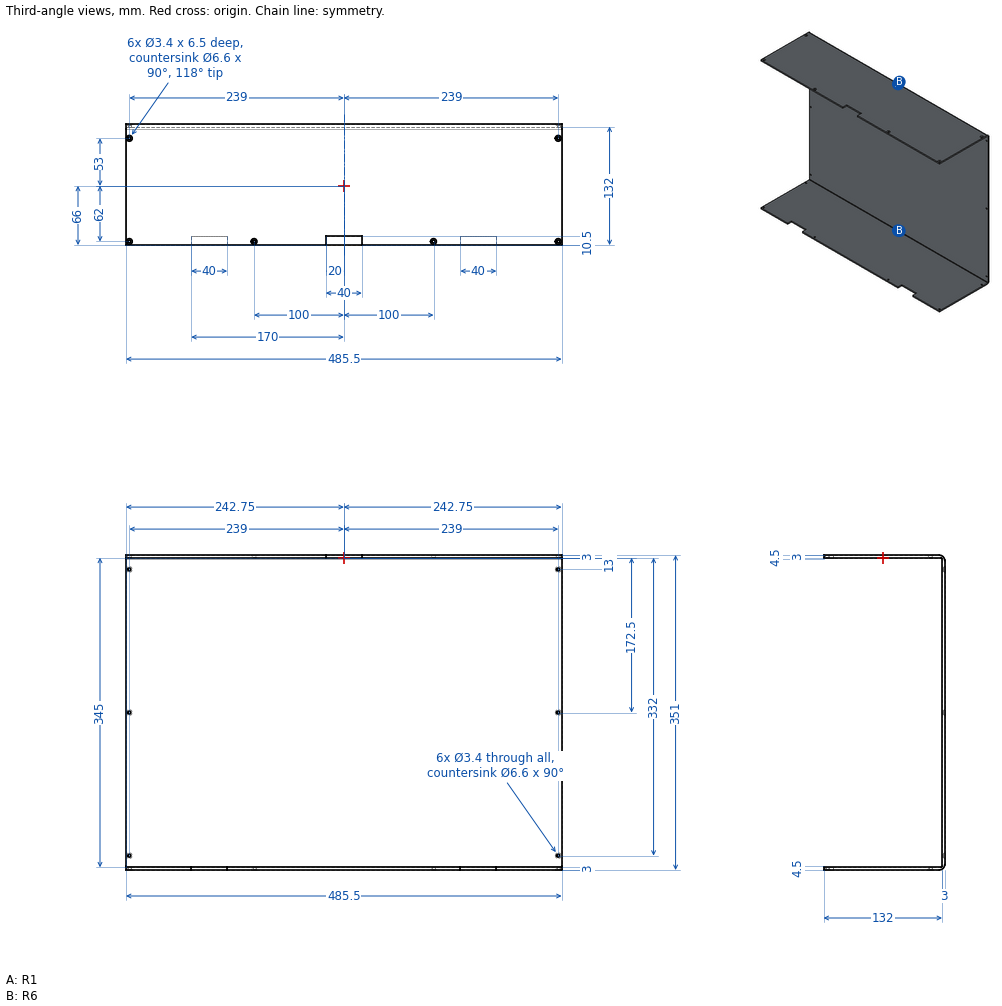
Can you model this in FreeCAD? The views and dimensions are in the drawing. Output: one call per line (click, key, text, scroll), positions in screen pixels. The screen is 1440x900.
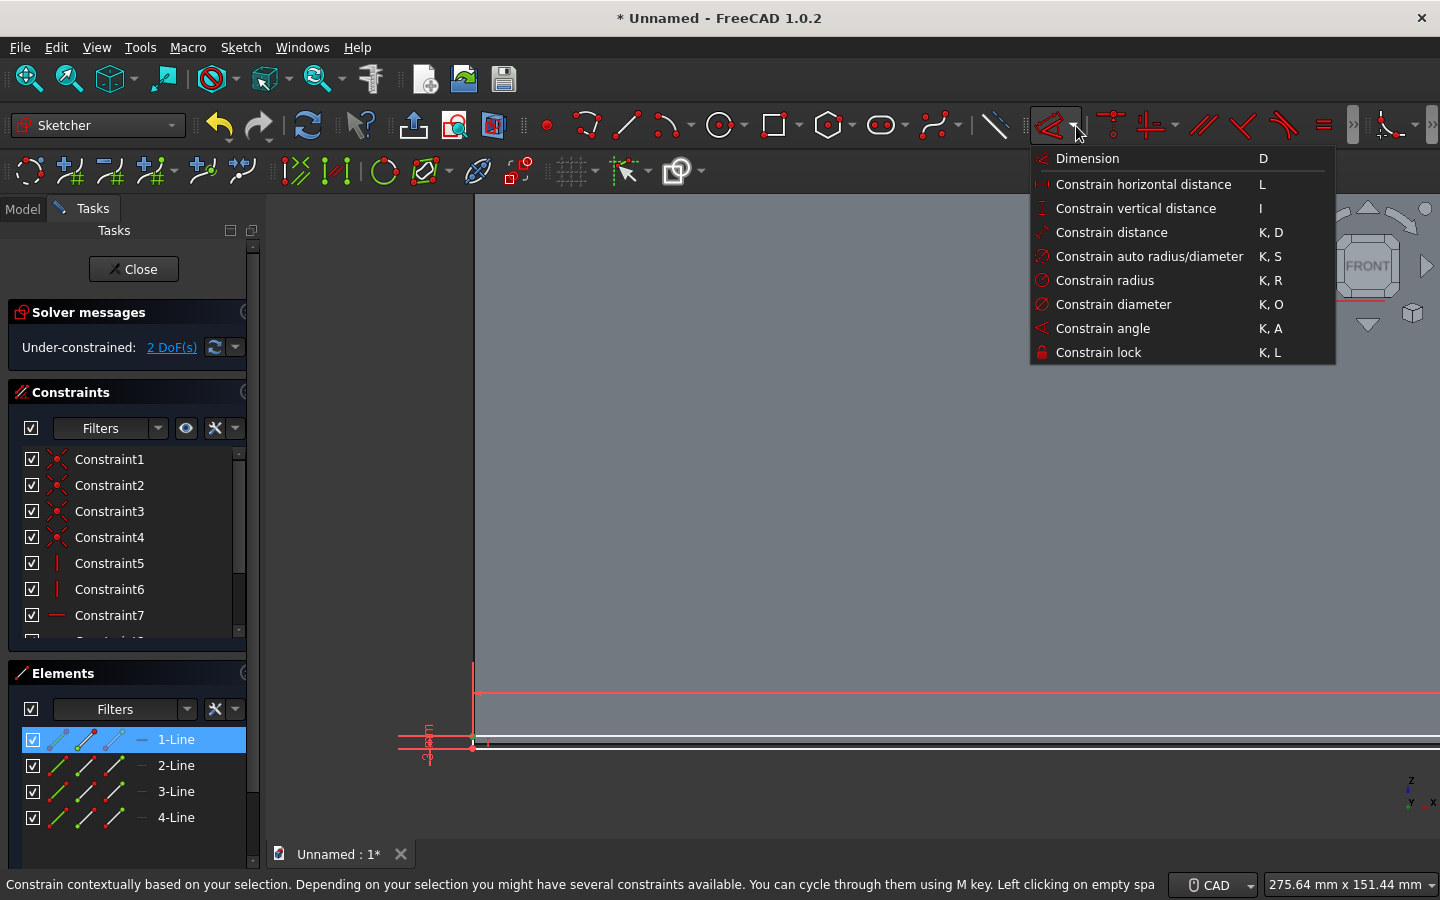
click(1183, 208)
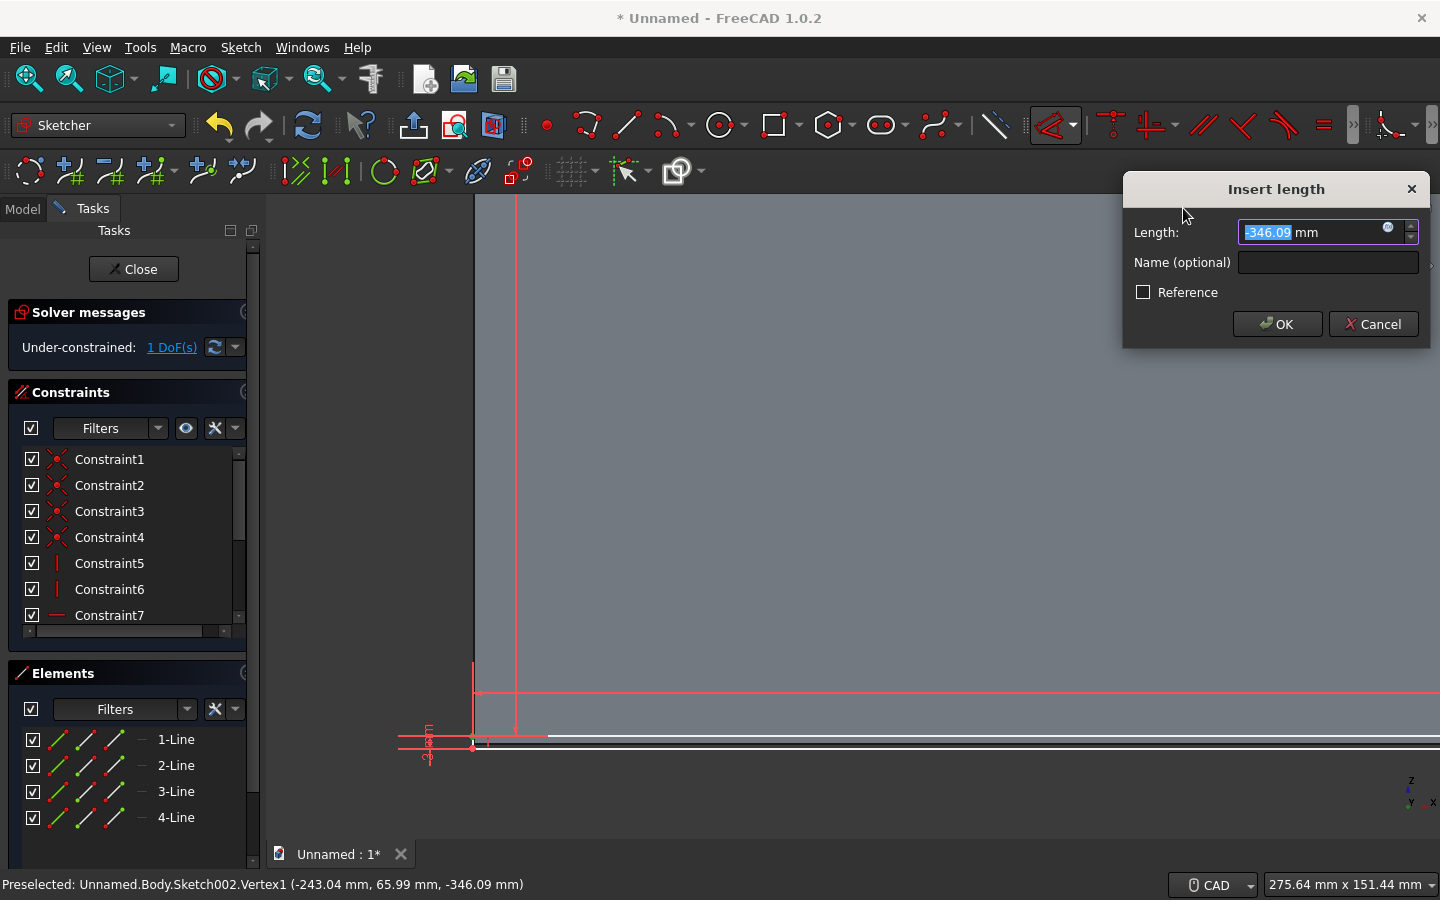
text(-345)
key(Return)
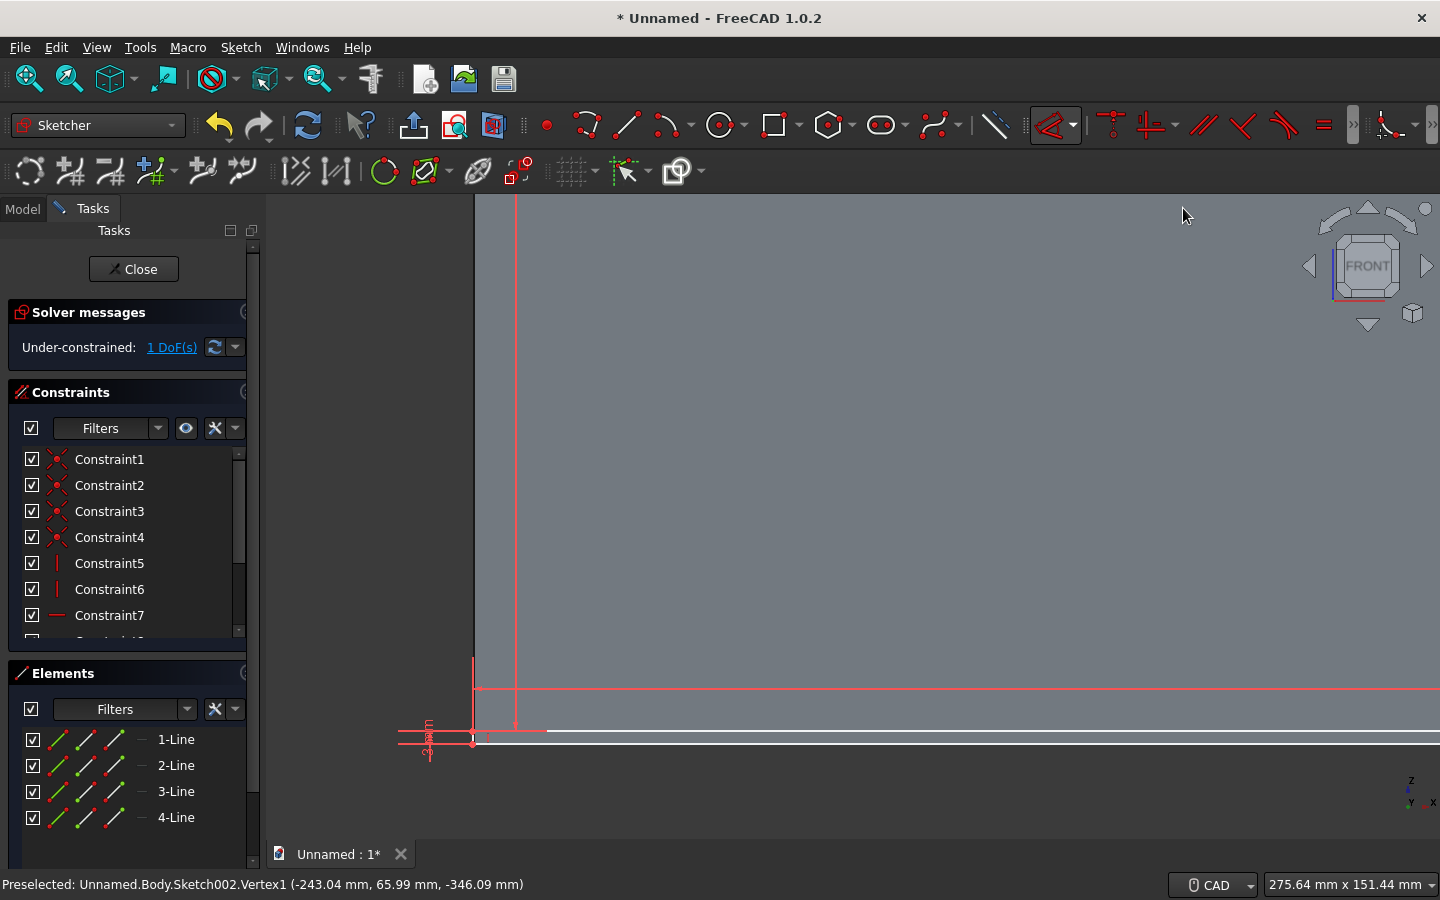
click(473, 731)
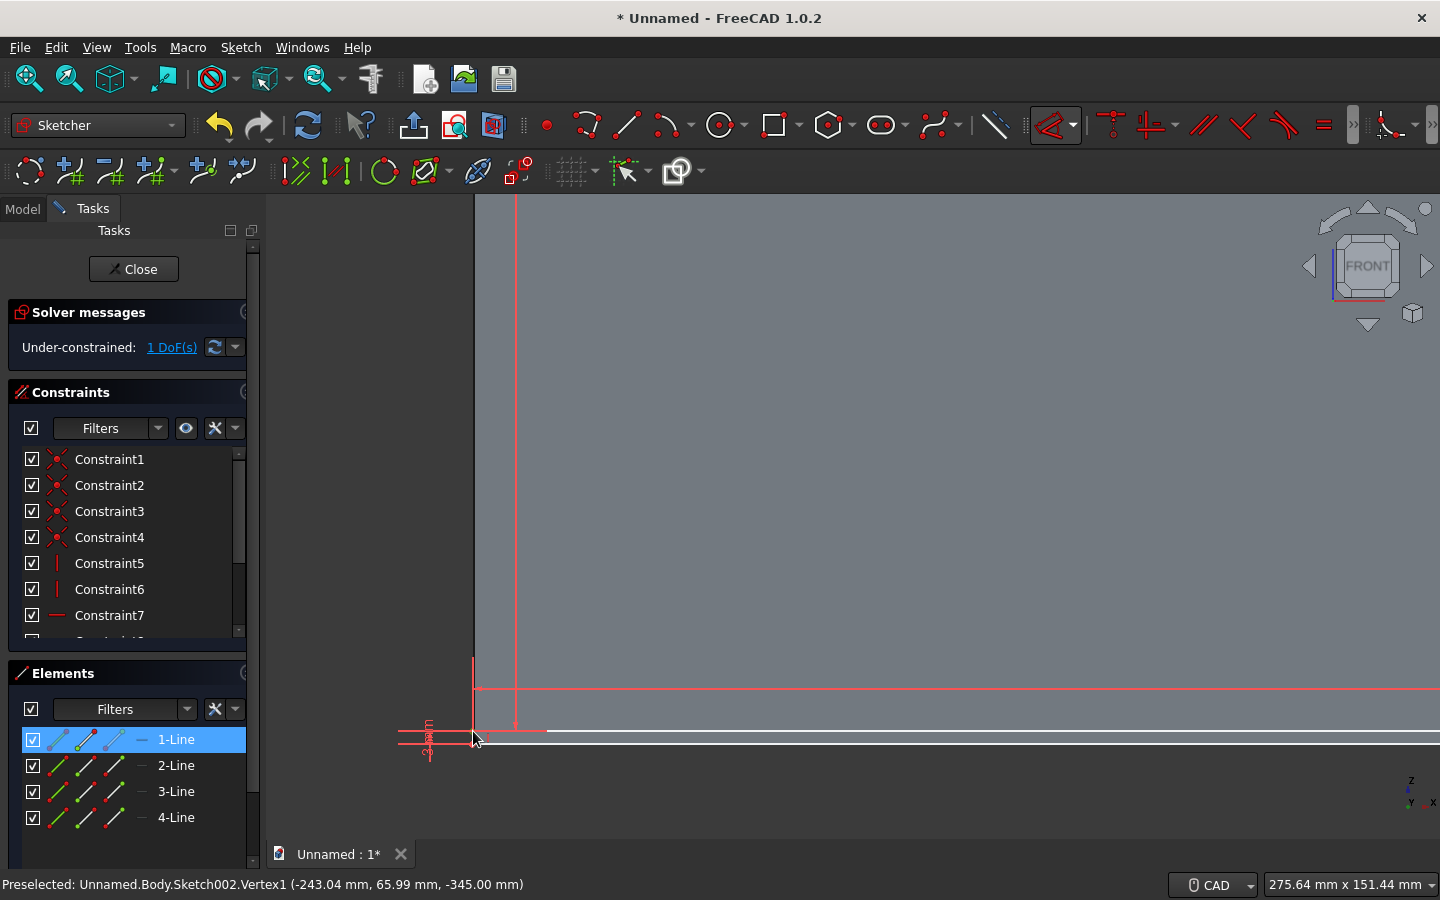
click(1076, 126)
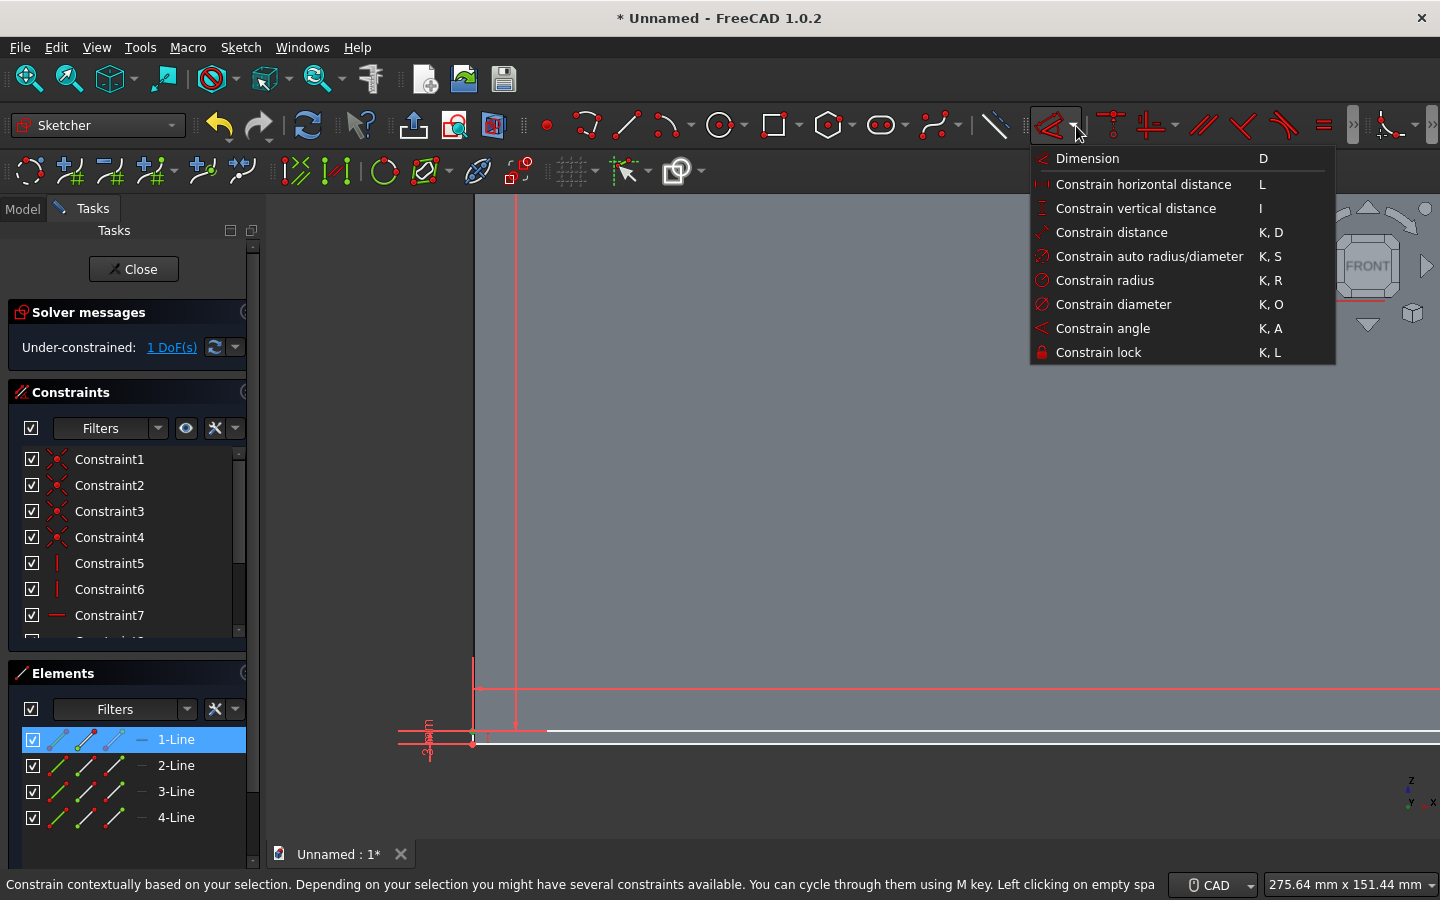
click(1183, 184)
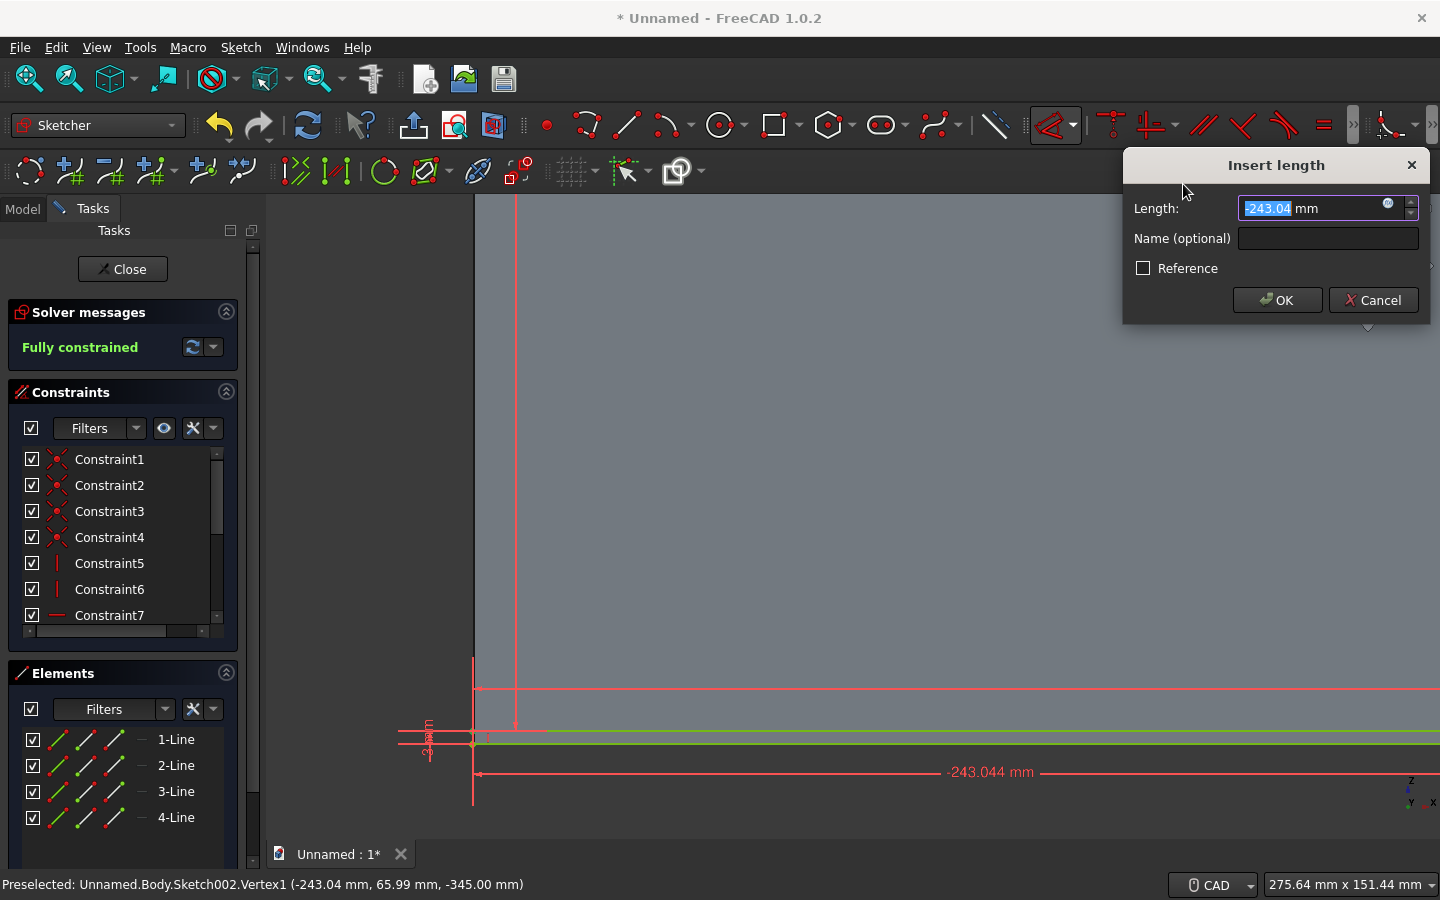
text(-242.75)
key(Return)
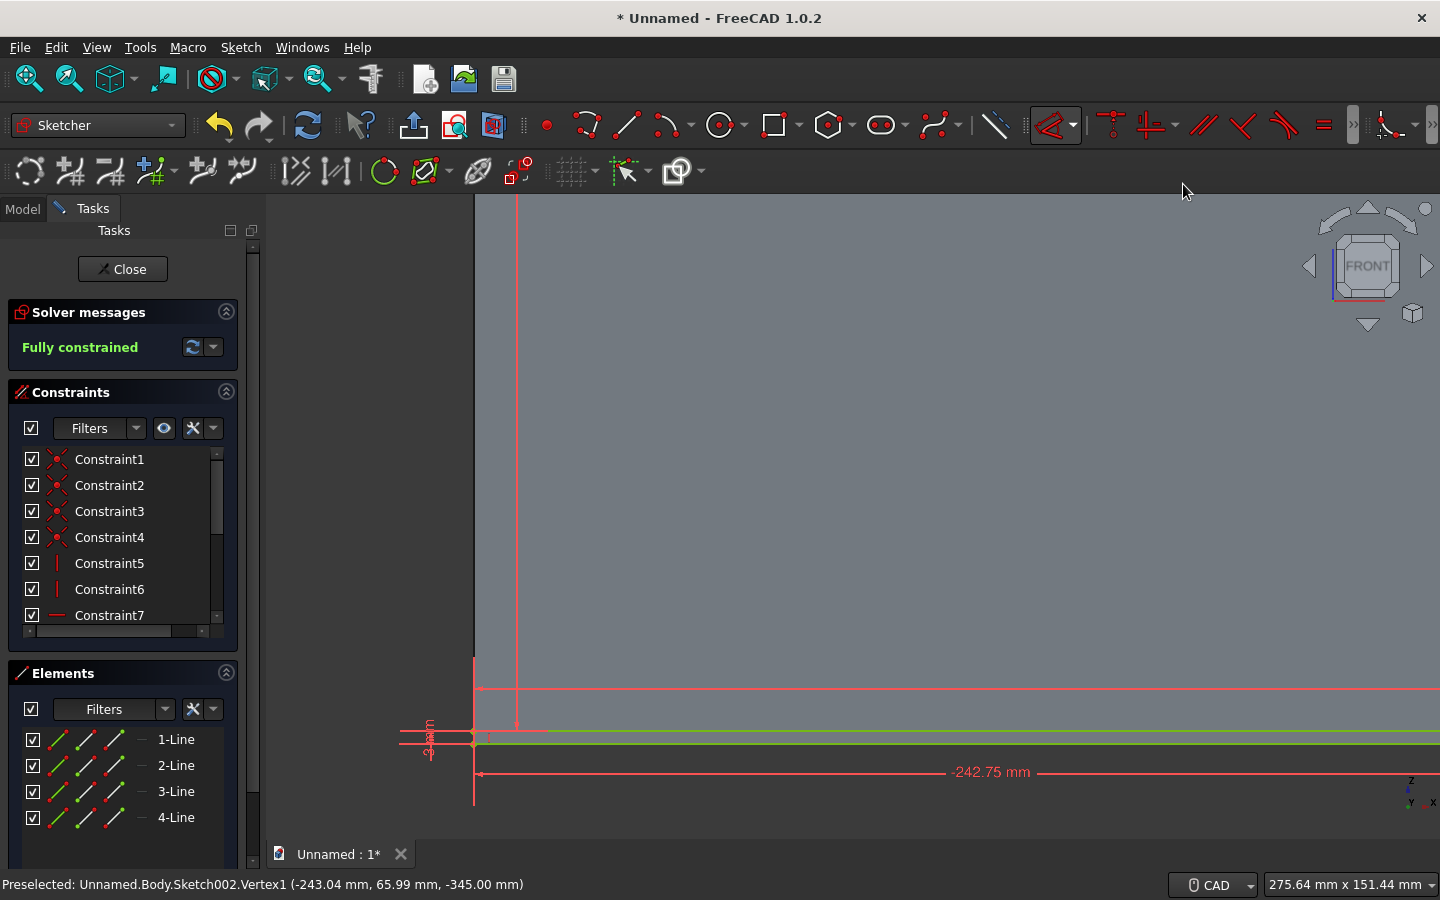
click(123, 269)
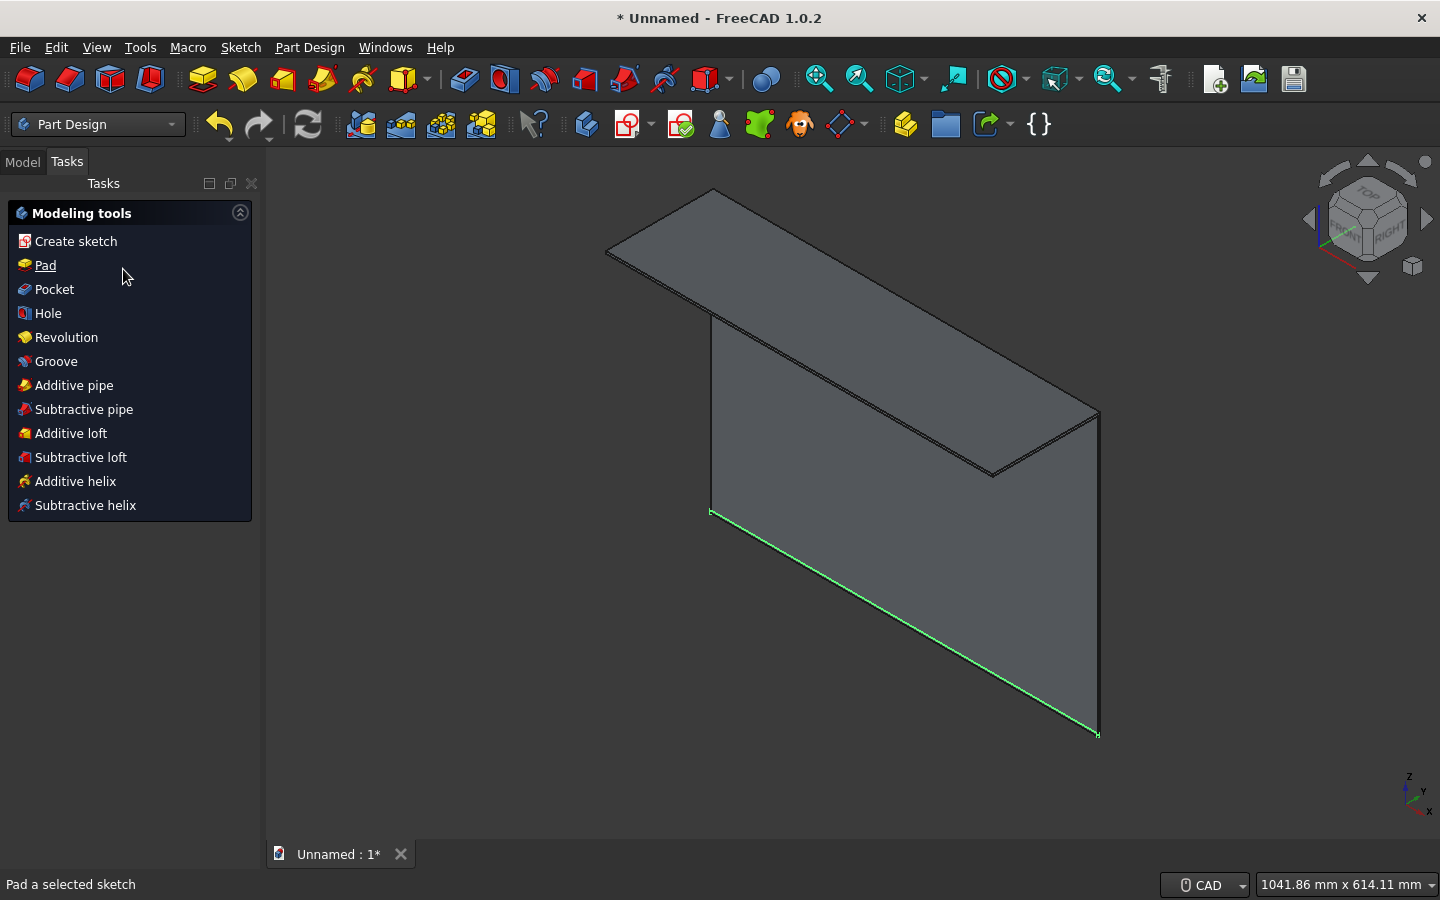
click(204, 80)